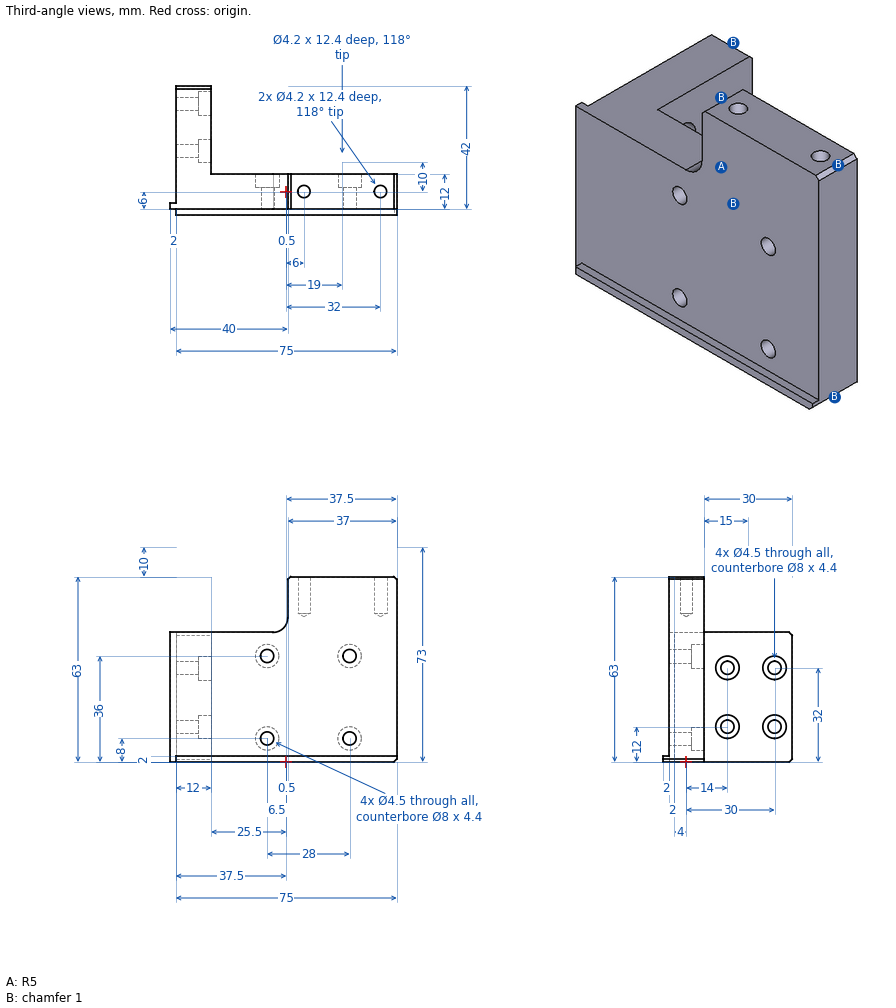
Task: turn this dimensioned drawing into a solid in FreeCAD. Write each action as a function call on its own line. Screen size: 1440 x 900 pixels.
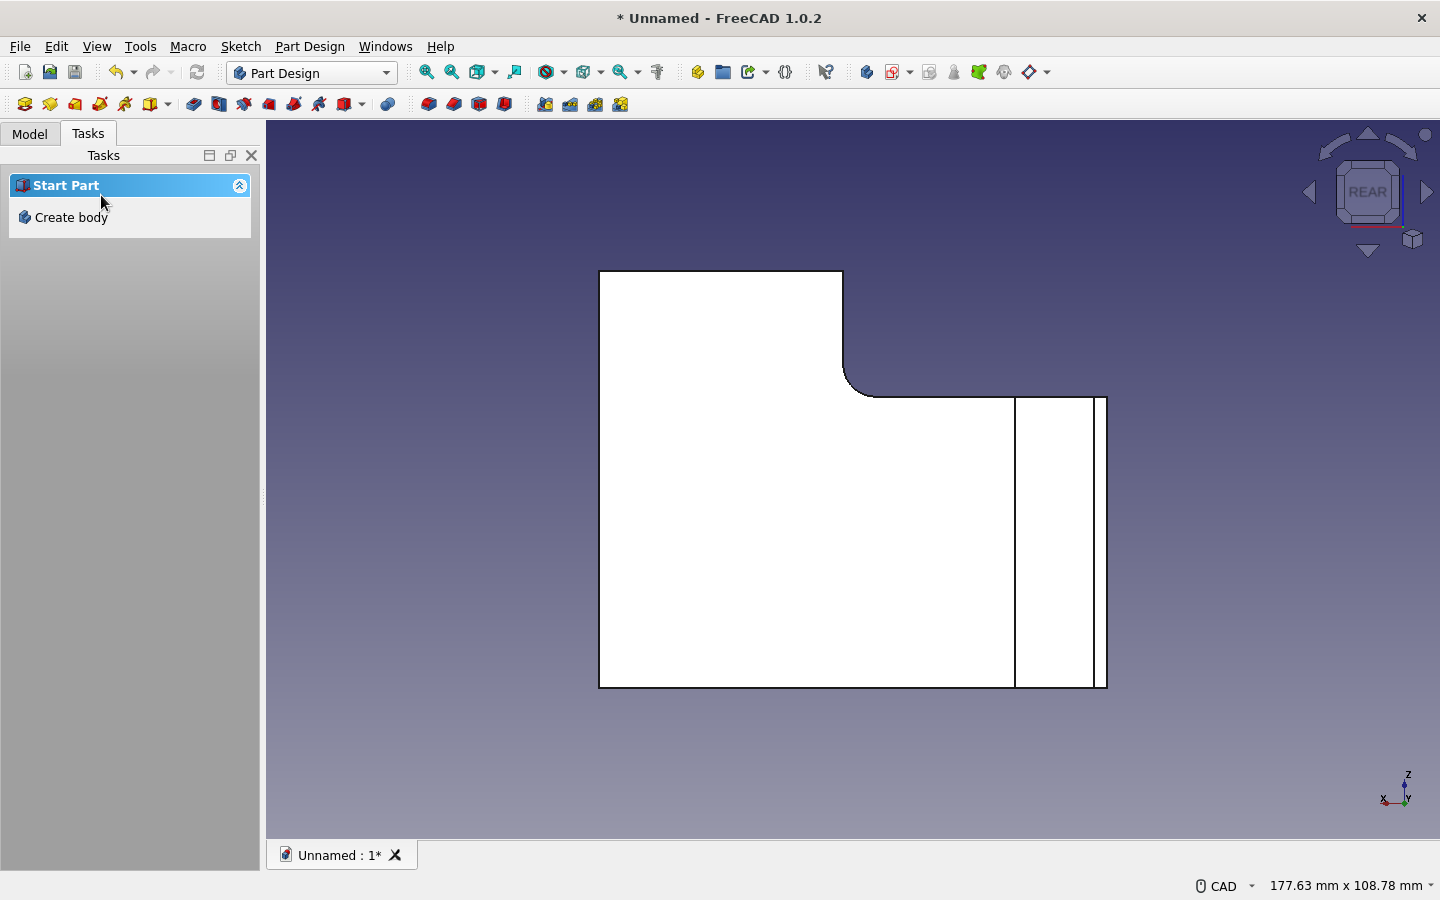
click(747, 538)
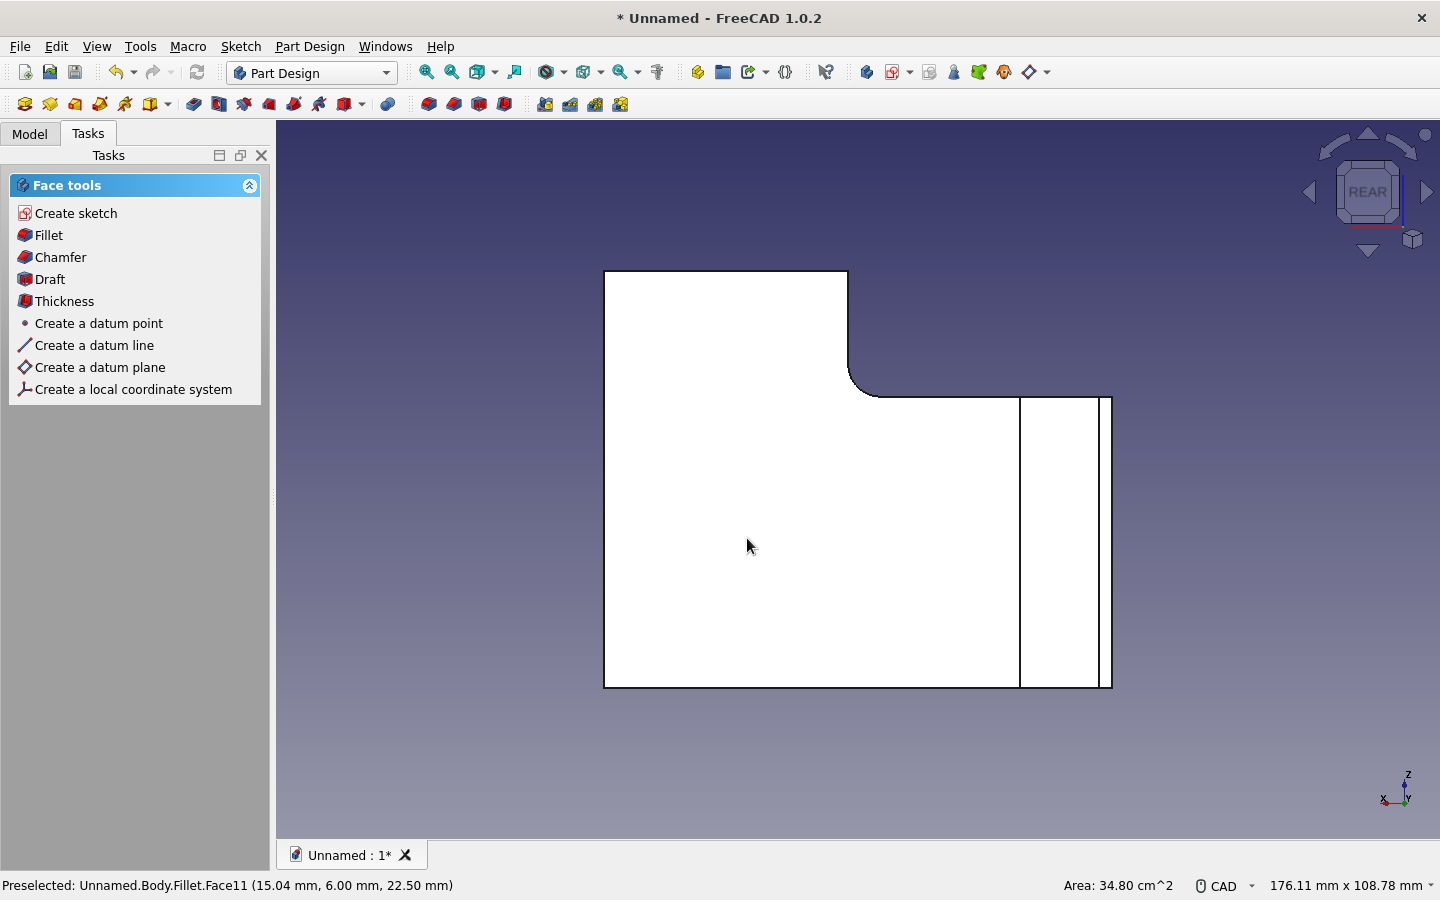
click(892, 72)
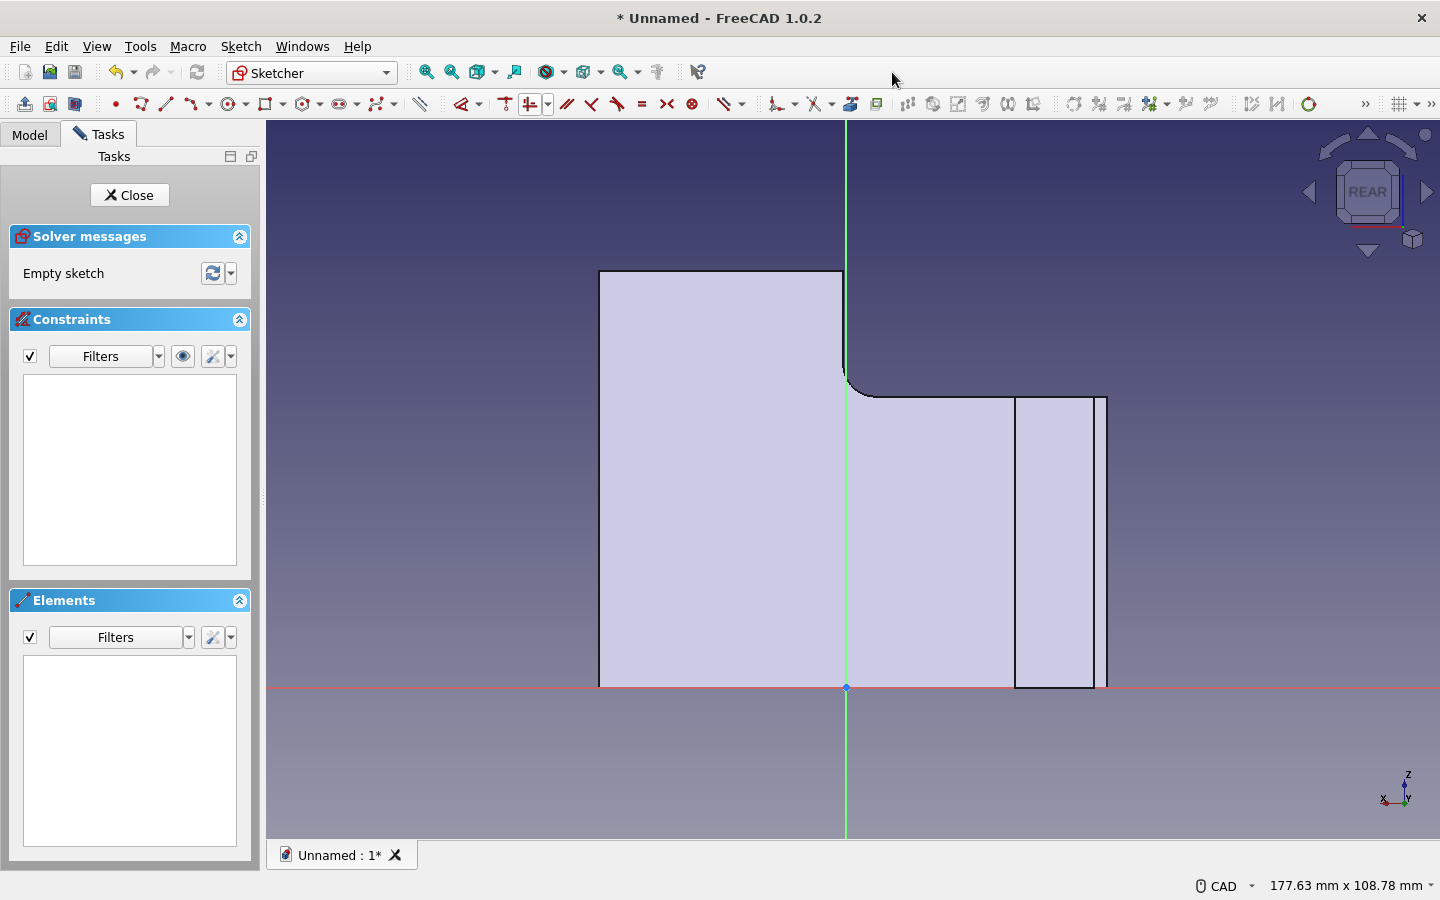
scroll(812, 661, up, 3)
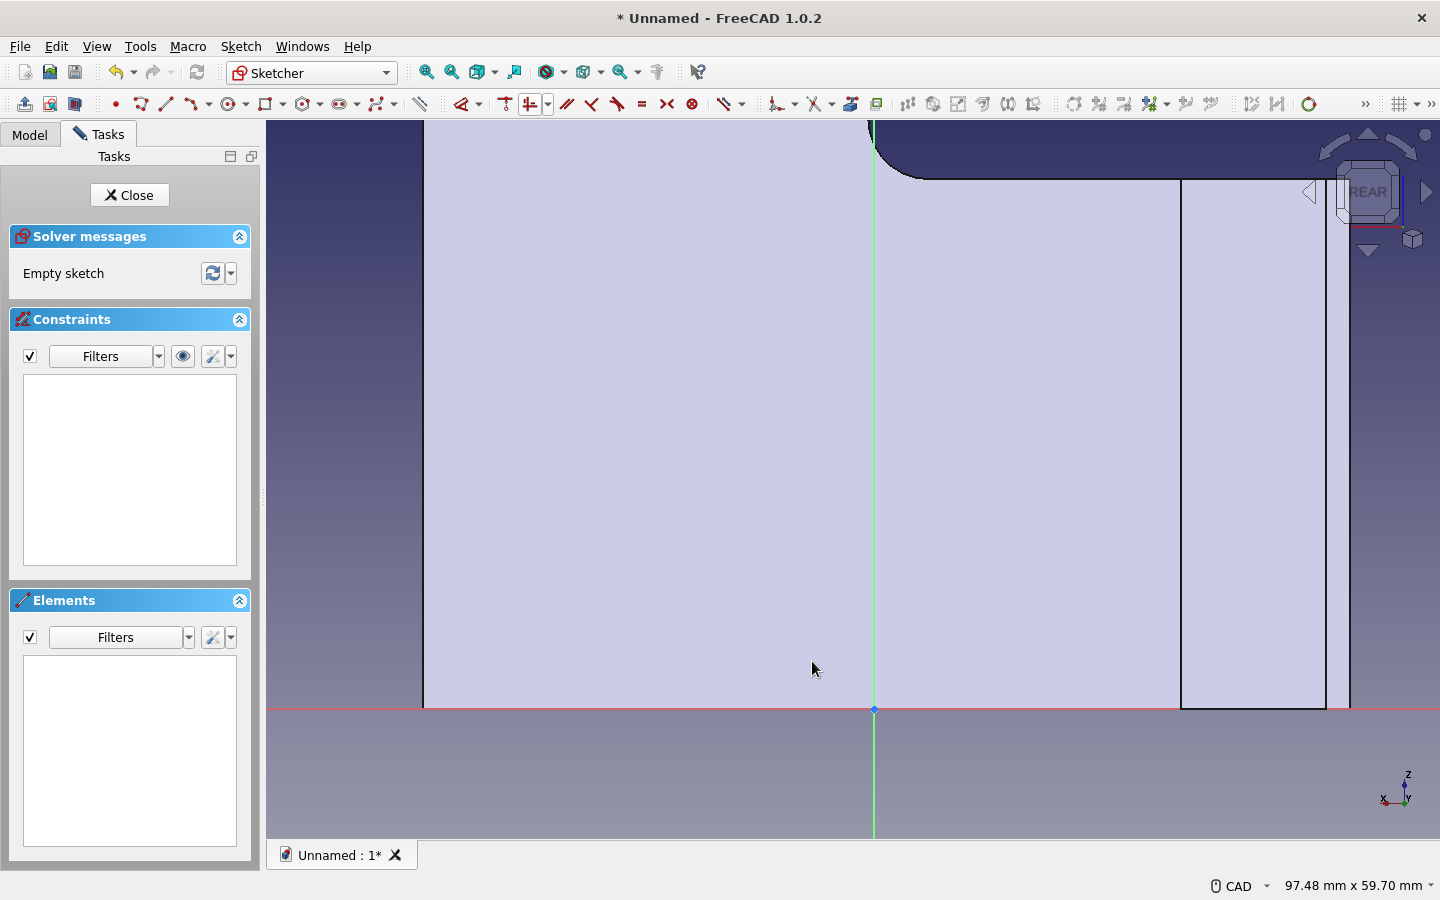
key(g)
key(c)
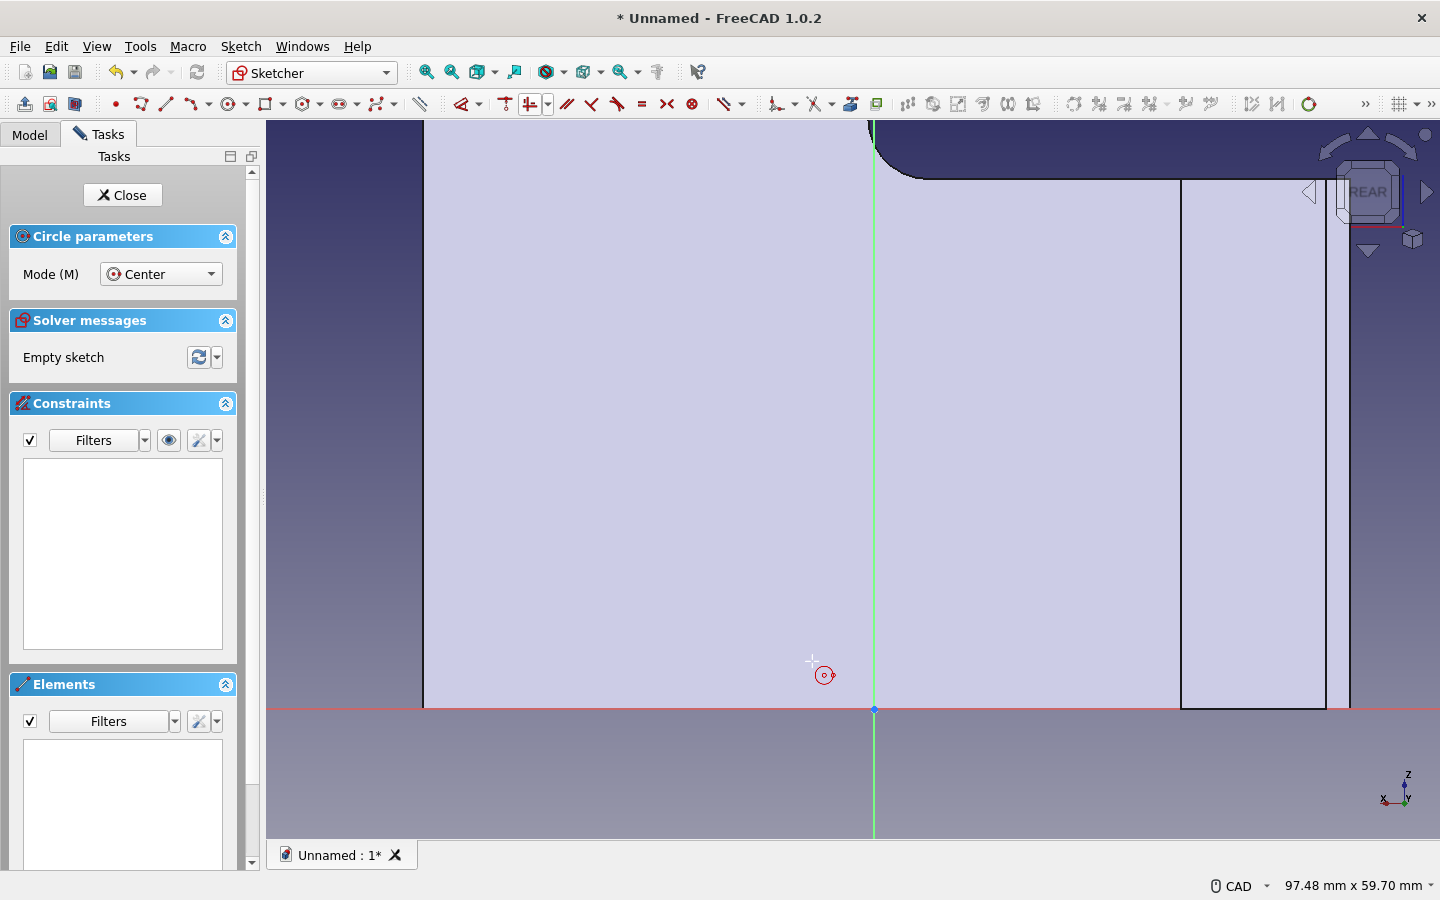
click(953, 613)
move(972, 594)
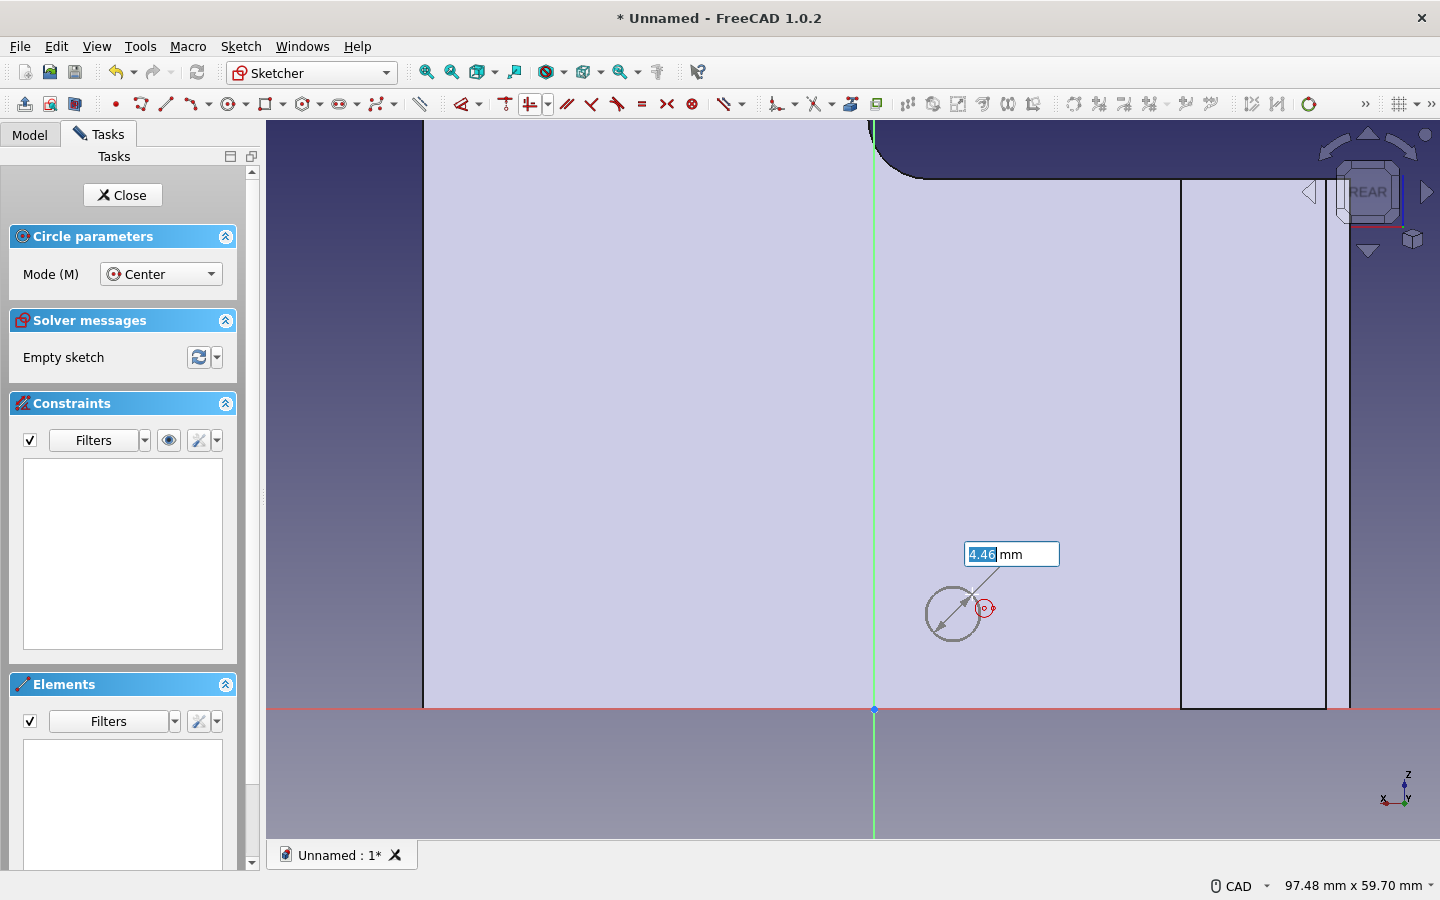
text(4.5)
key(Return)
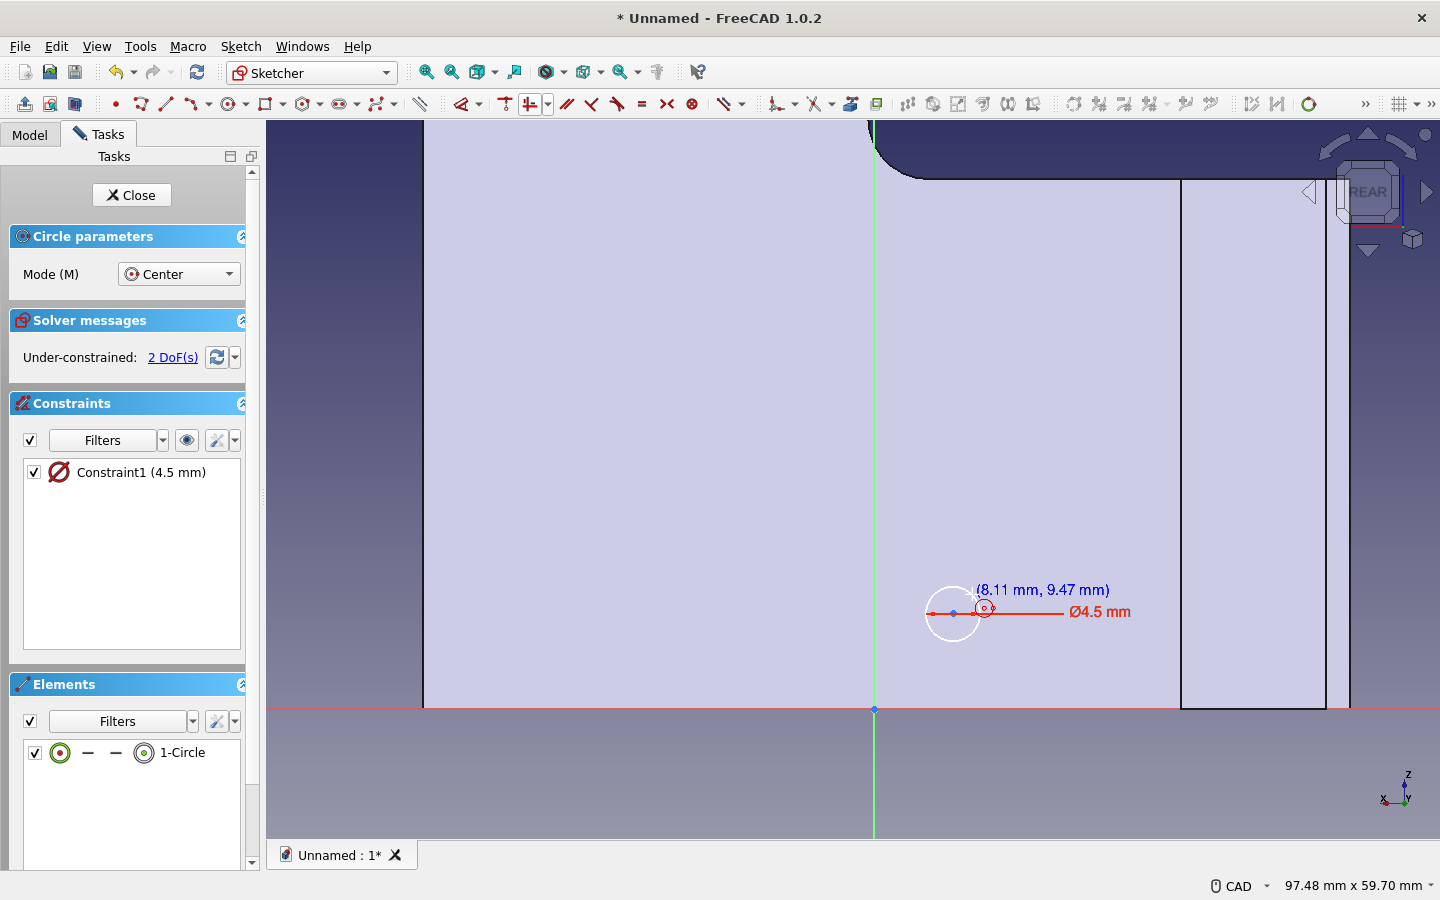
click(615, 613)
move(635, 594)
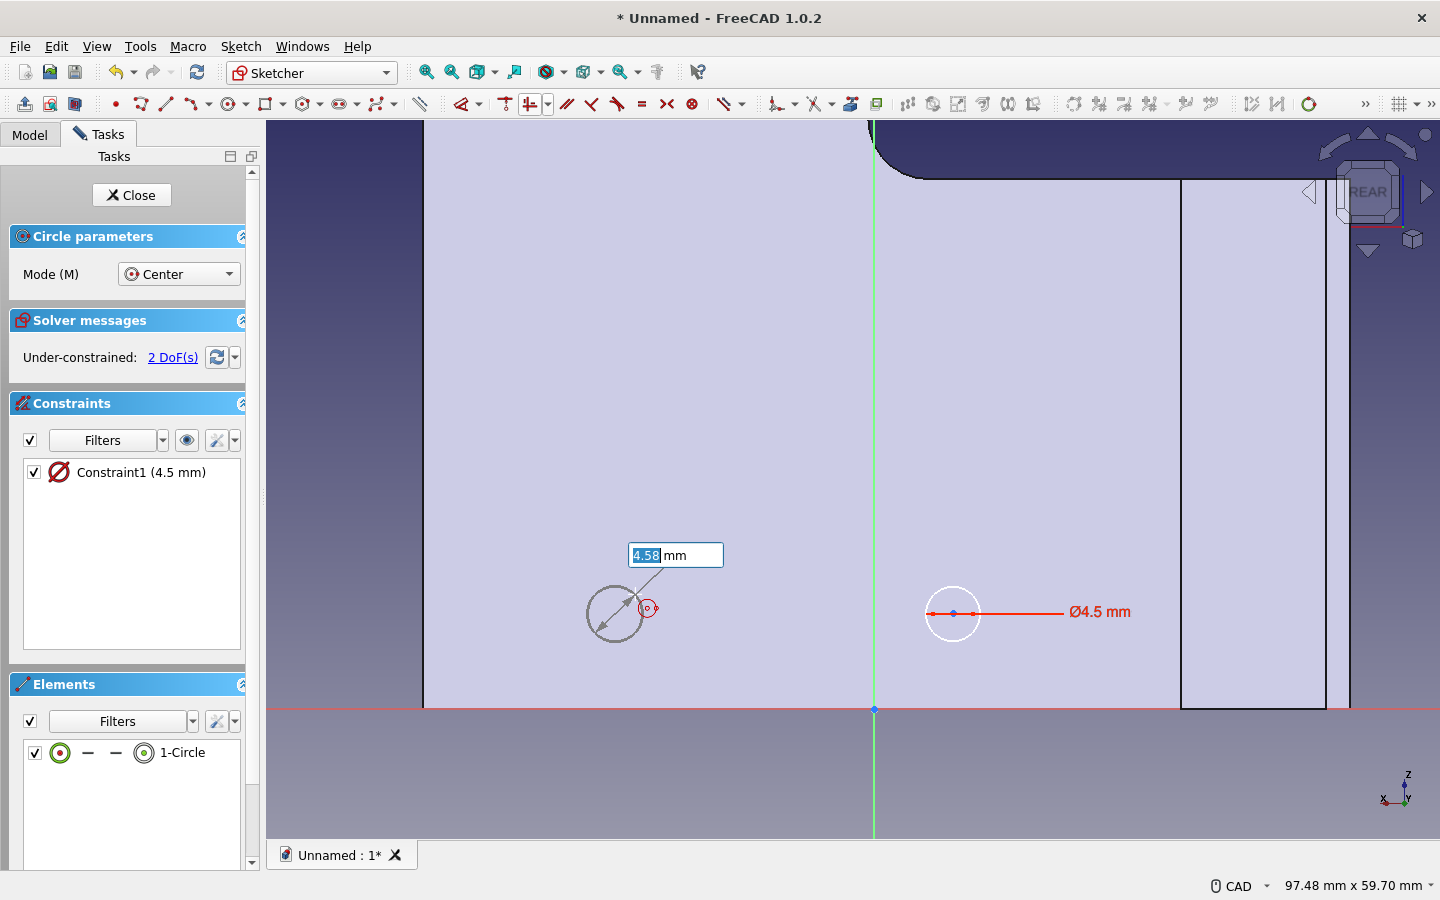
text(4.5)
key(Return)